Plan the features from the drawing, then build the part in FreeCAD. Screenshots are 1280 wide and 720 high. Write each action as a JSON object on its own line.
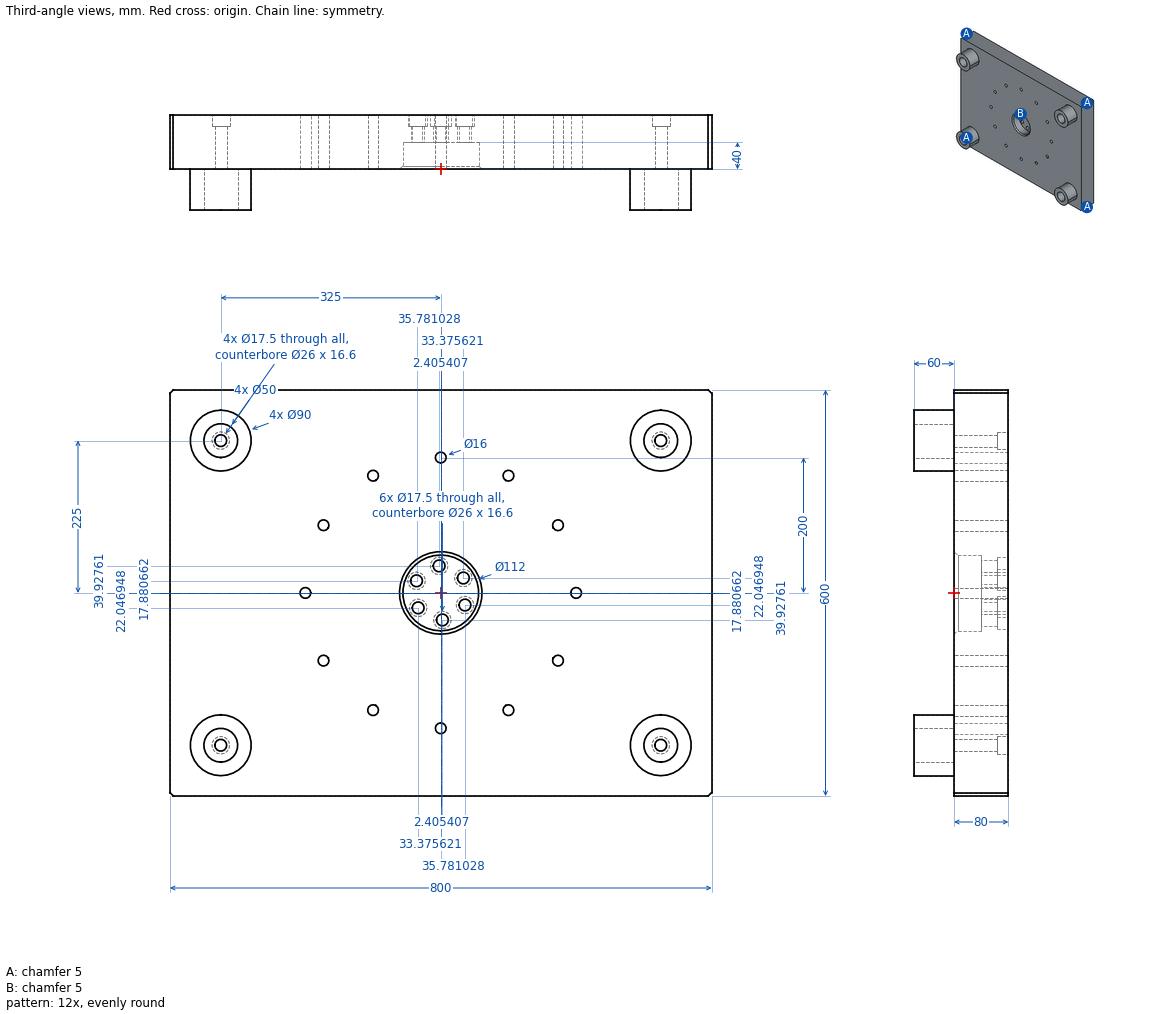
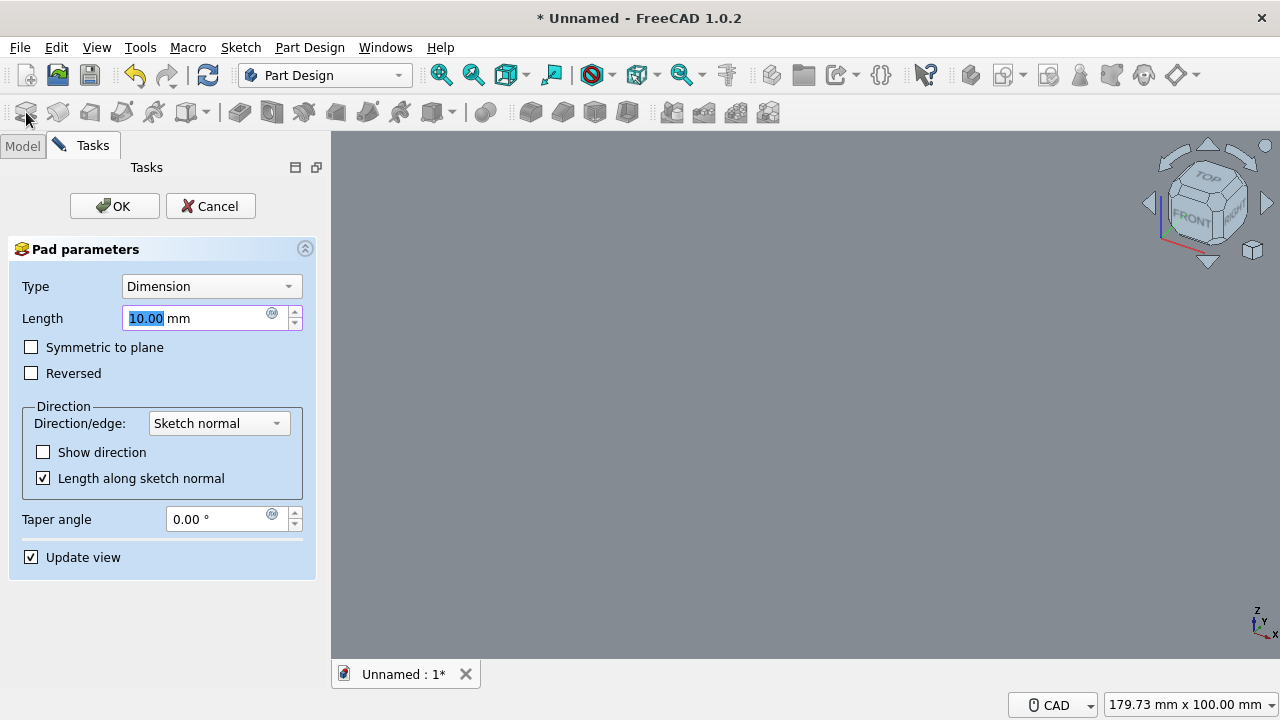
{"action": "type", "text": "80"}
{"action": "key", "text": "Tab"}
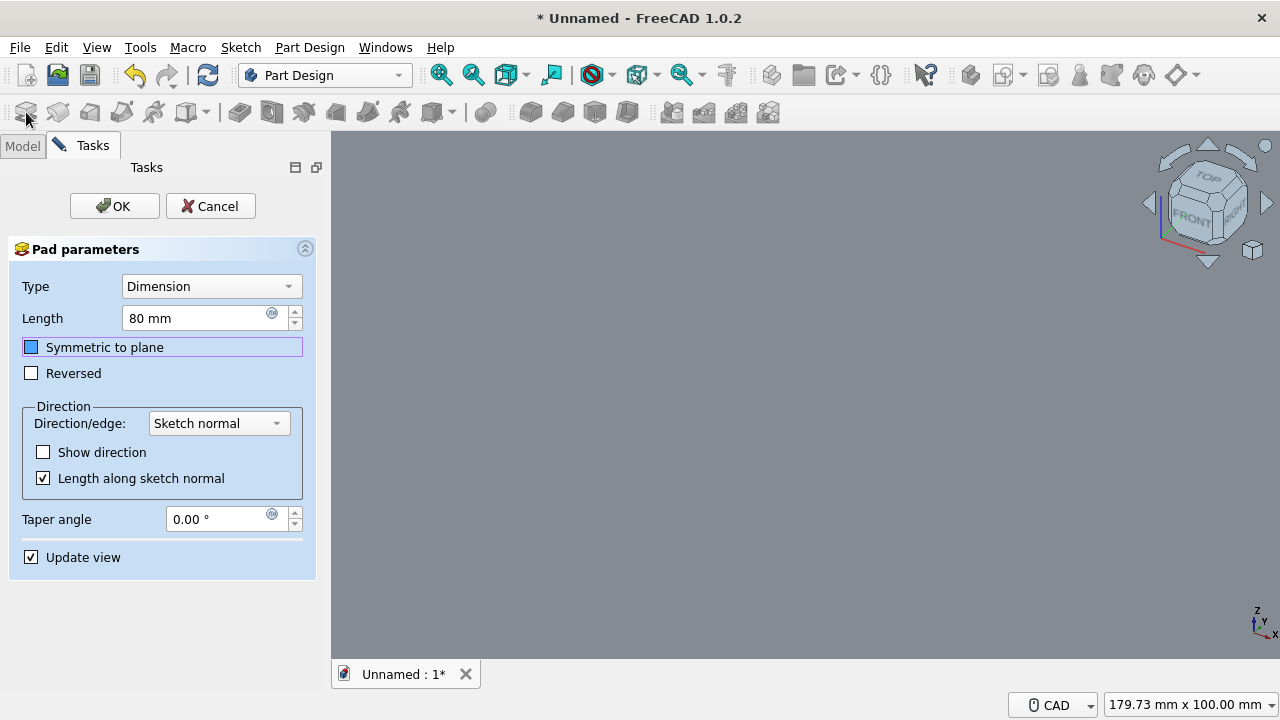
{"action": "left_click", "coordinate": [30, 373]}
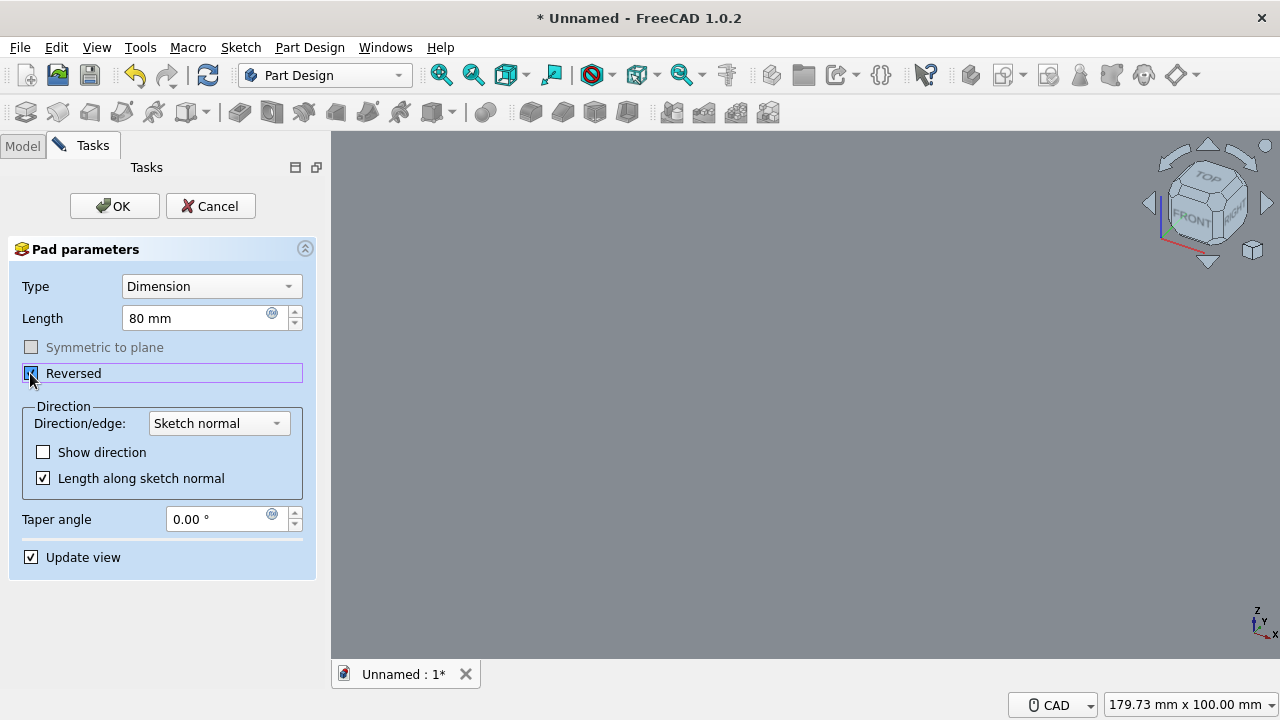
{"action": "left_click", "coordinate": [115, 206]}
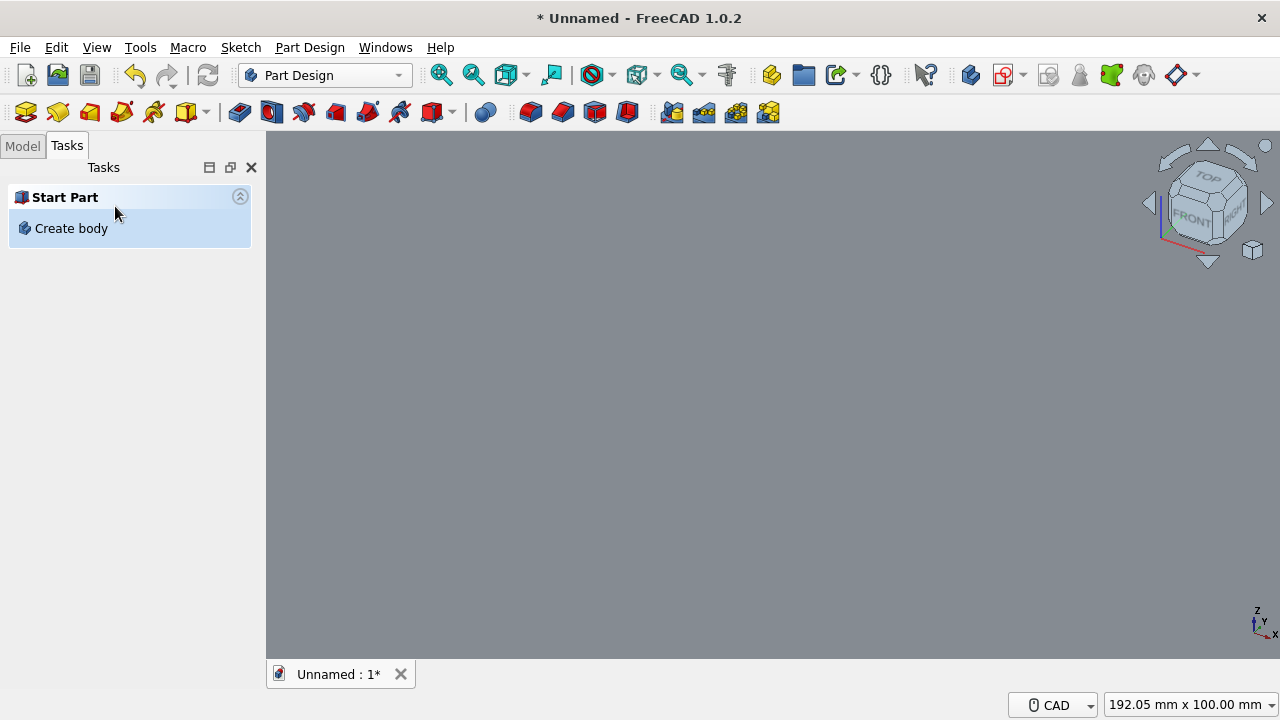
{"action": "key", "text": "v f"}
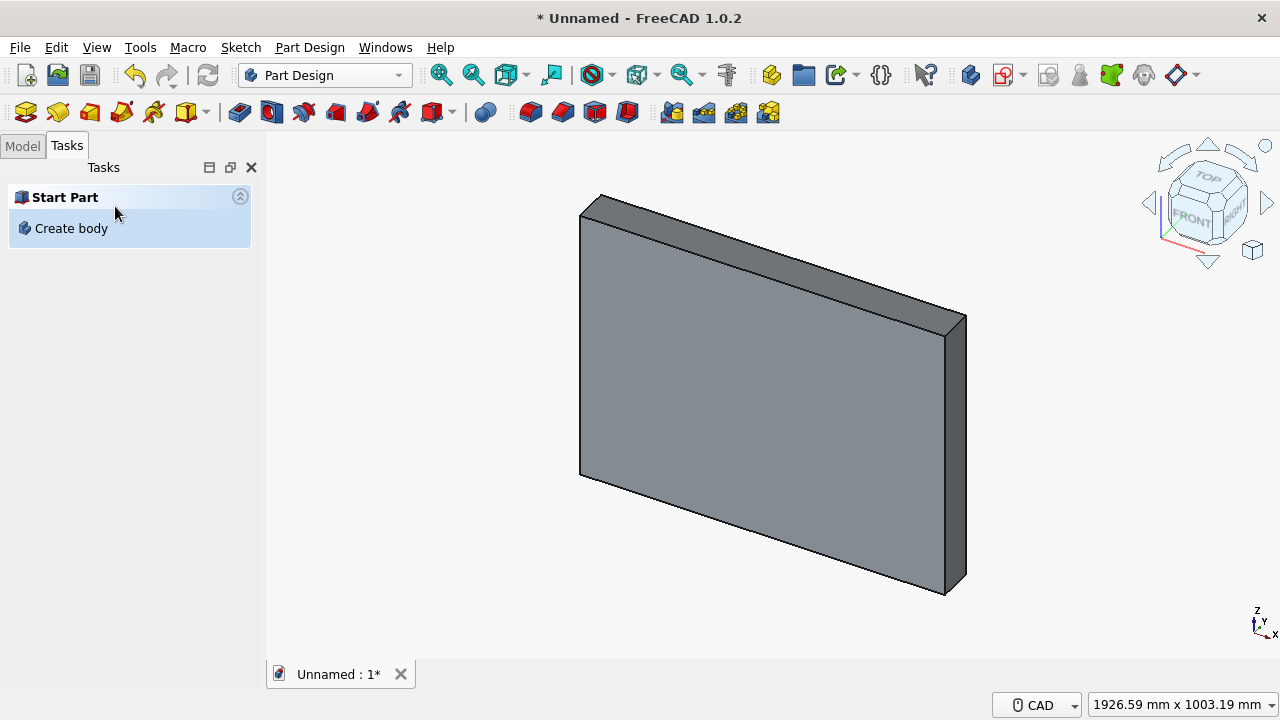
{"action": "left_click", "coordinate": [955, 325]}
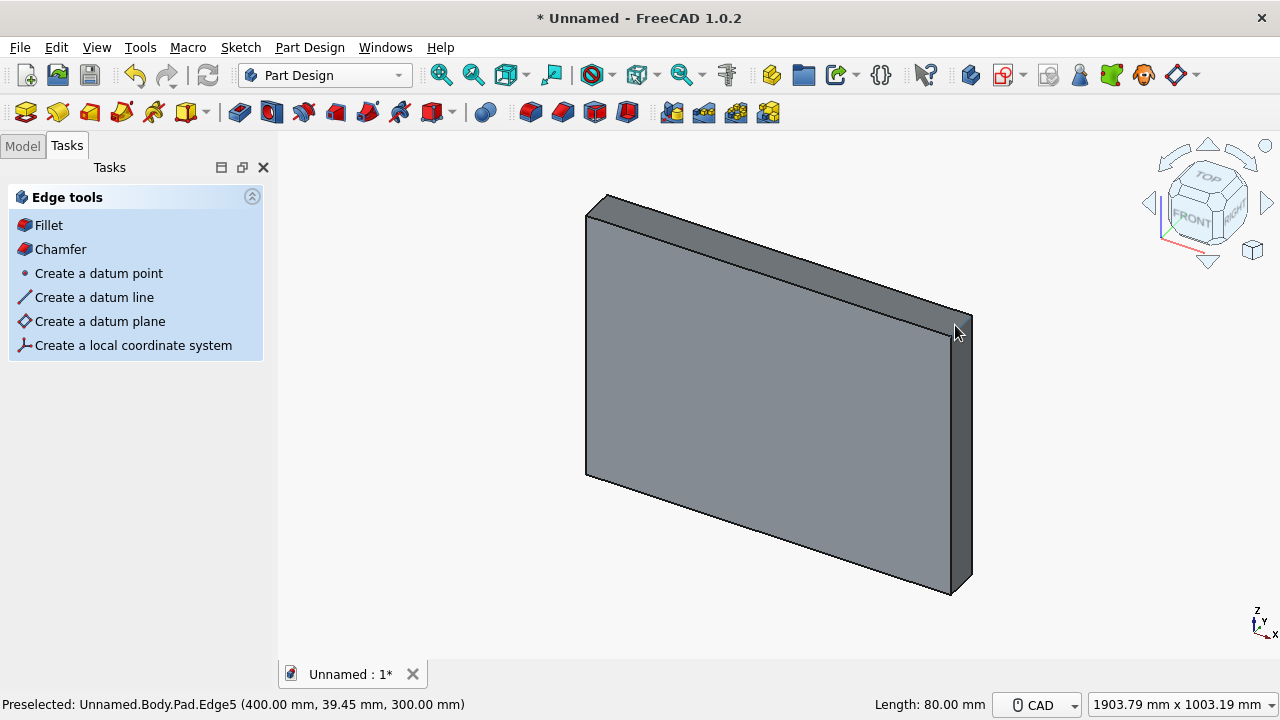
{"action": "key", "text": "0"}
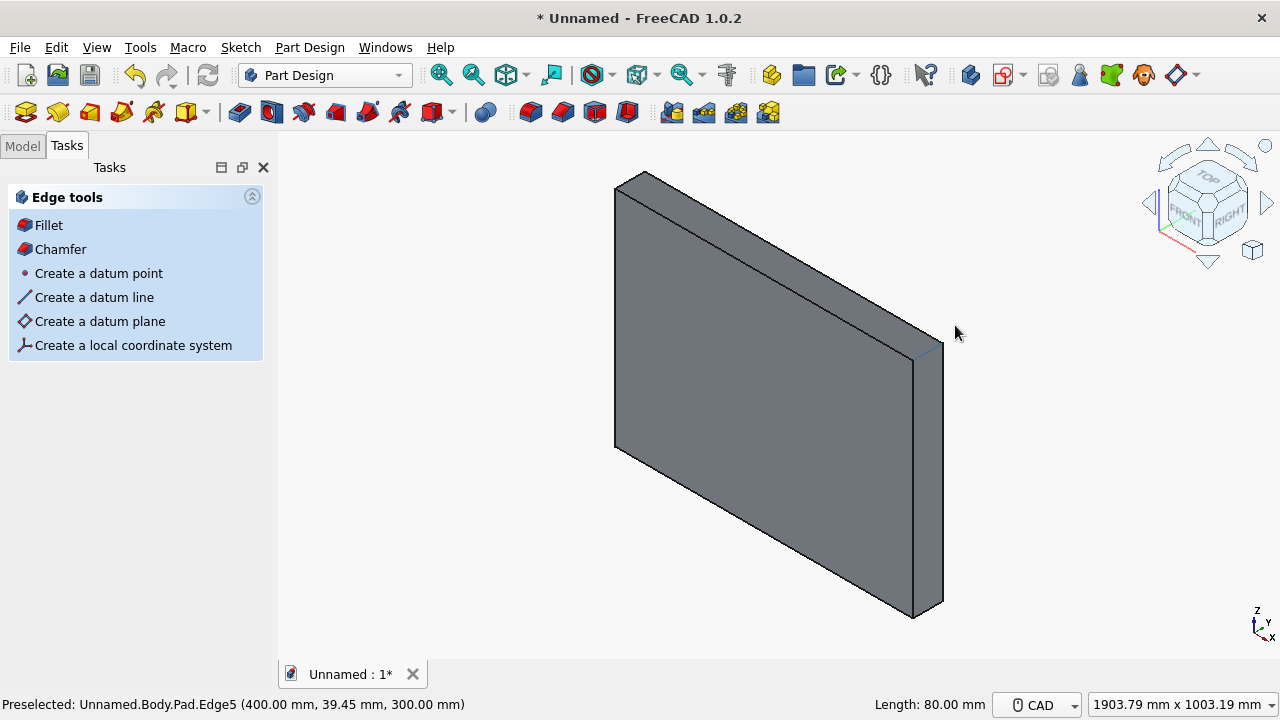
{"action": "key", "text": "2"}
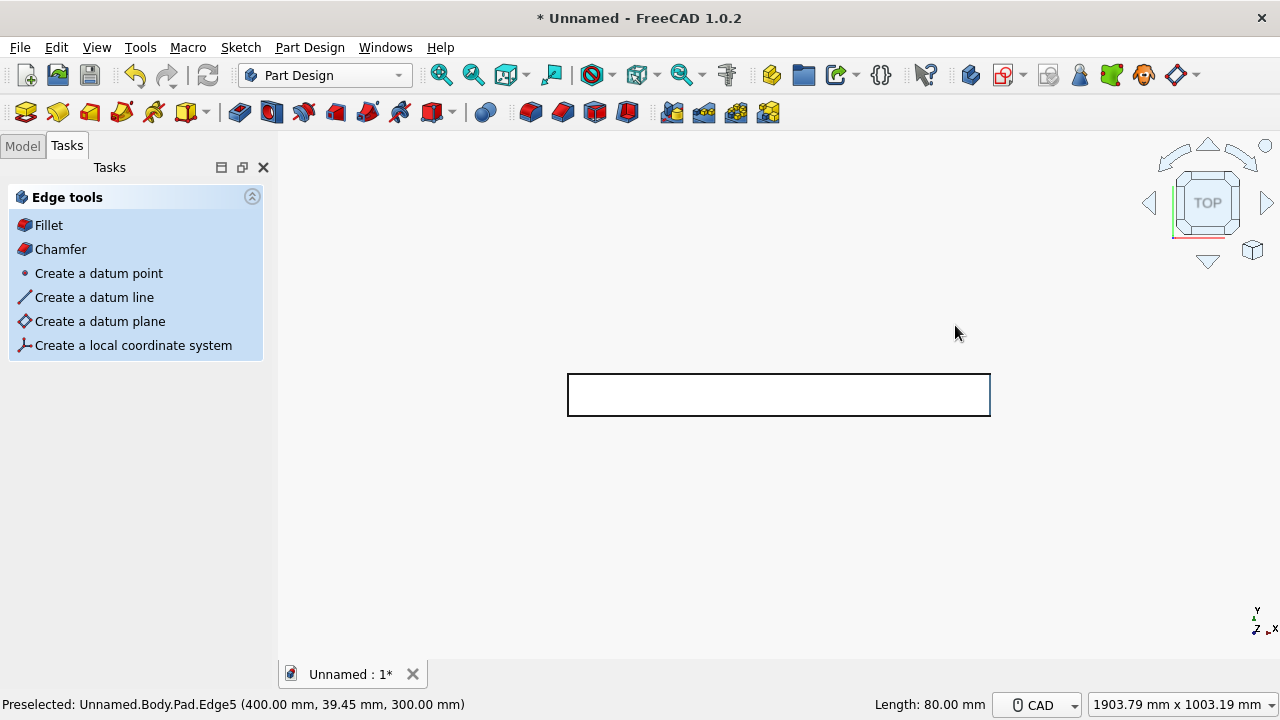
{"action": "key", "text": "v f"}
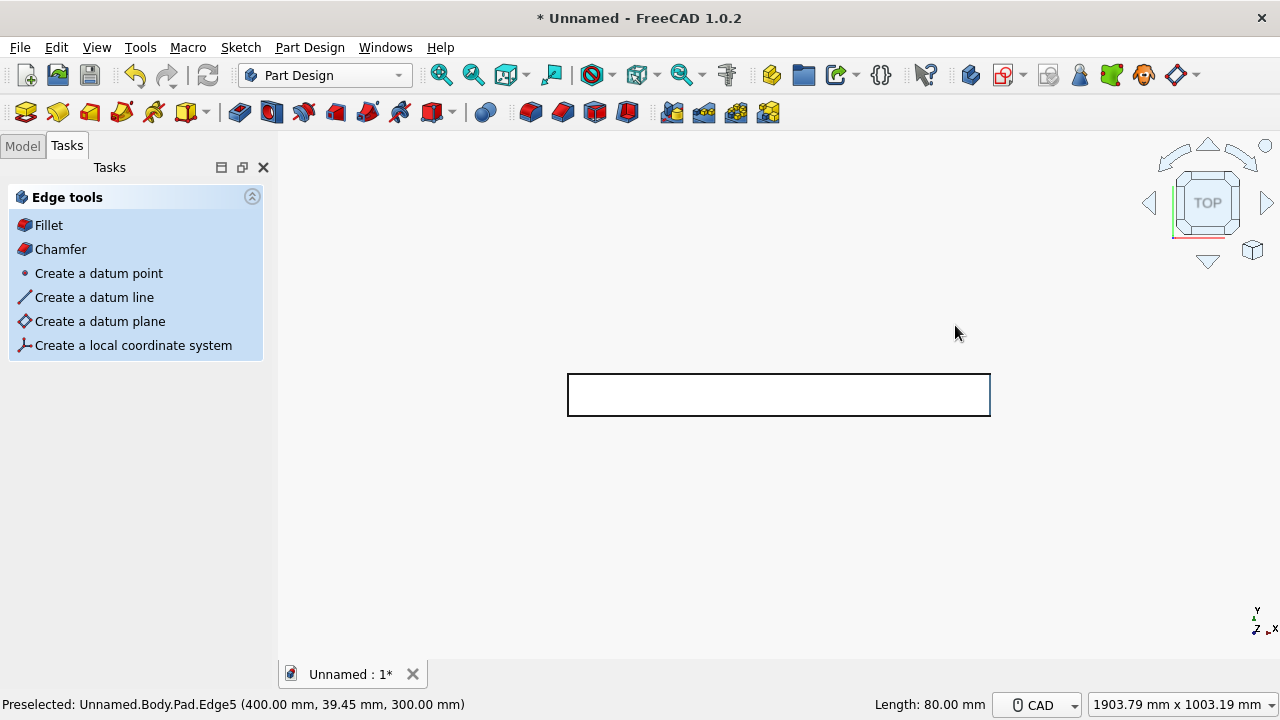
{"action": "left_click", "coordinate": [568, 394], "text": "ctrl"}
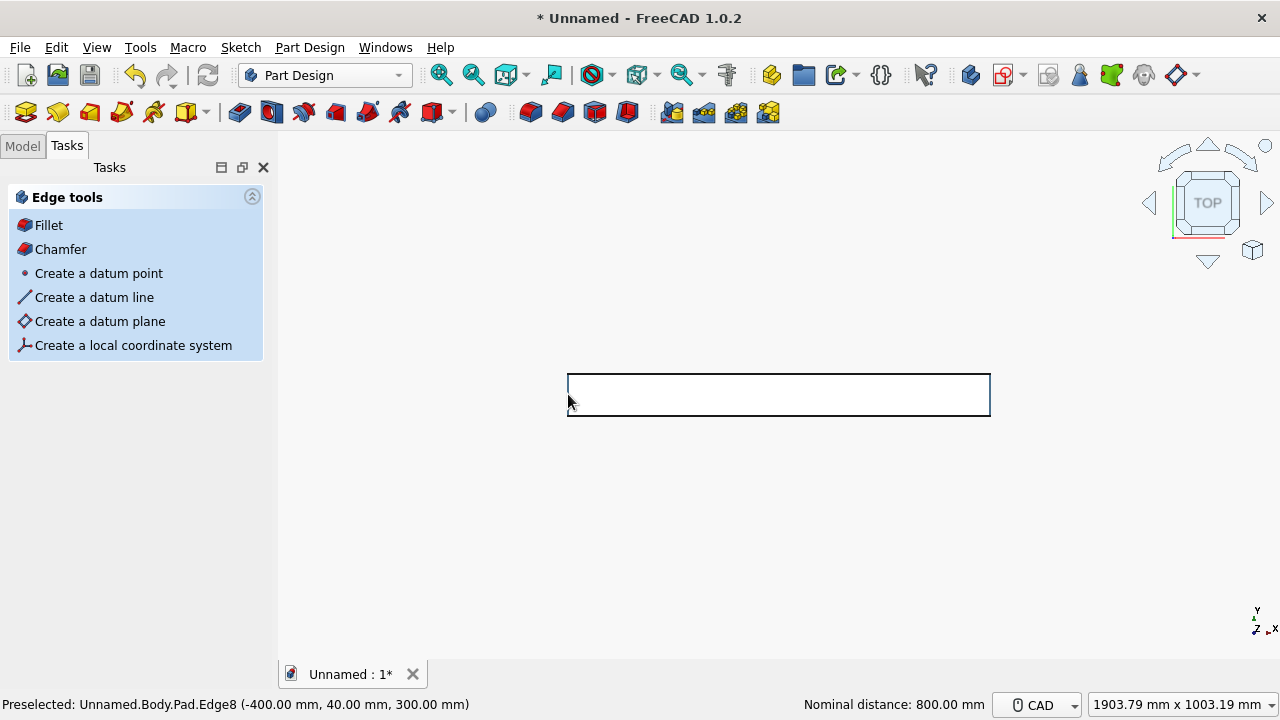
{"action": "key", "text": "1"}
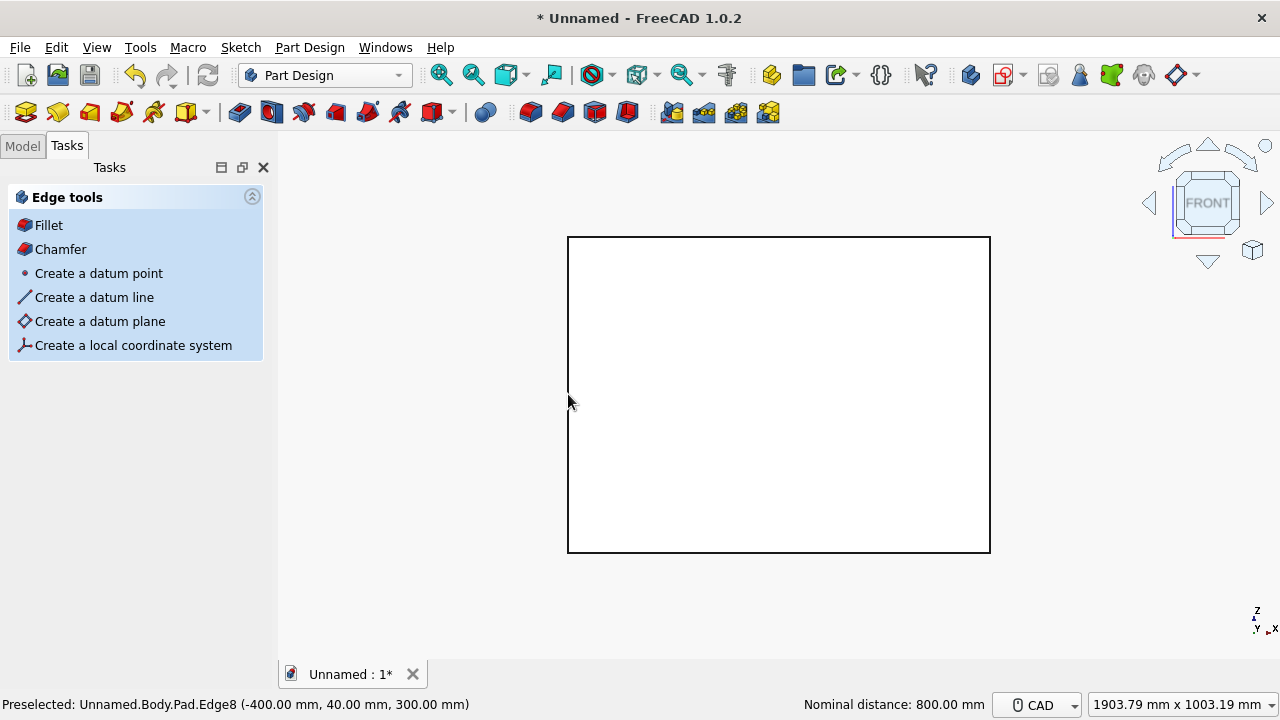
{"action": "key", "text": "3"}